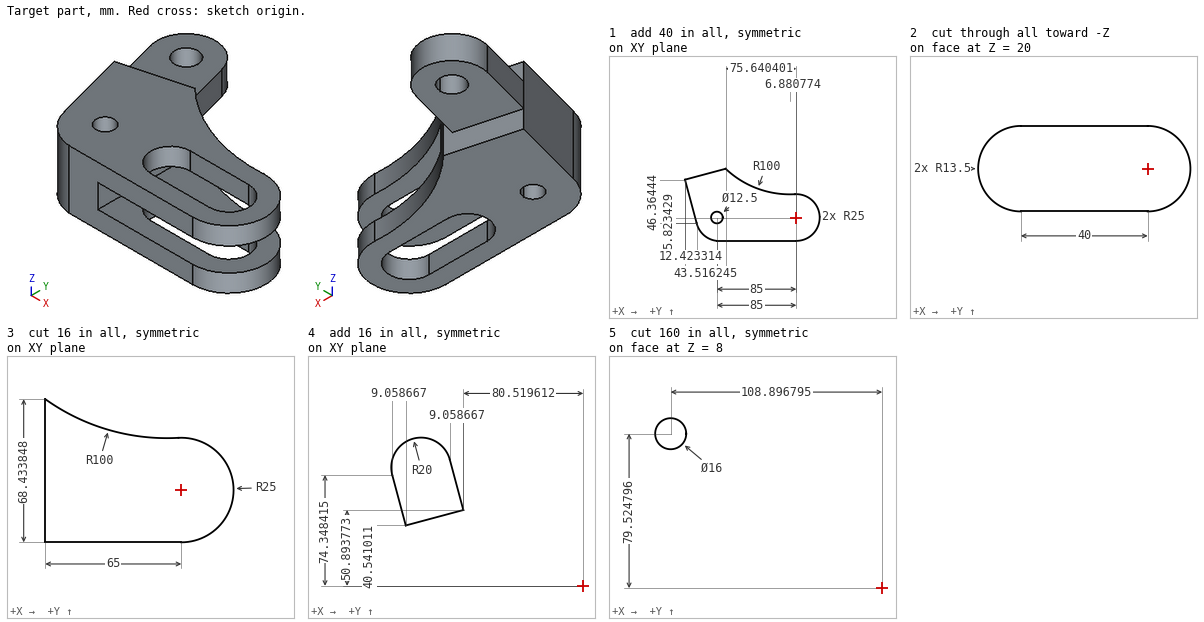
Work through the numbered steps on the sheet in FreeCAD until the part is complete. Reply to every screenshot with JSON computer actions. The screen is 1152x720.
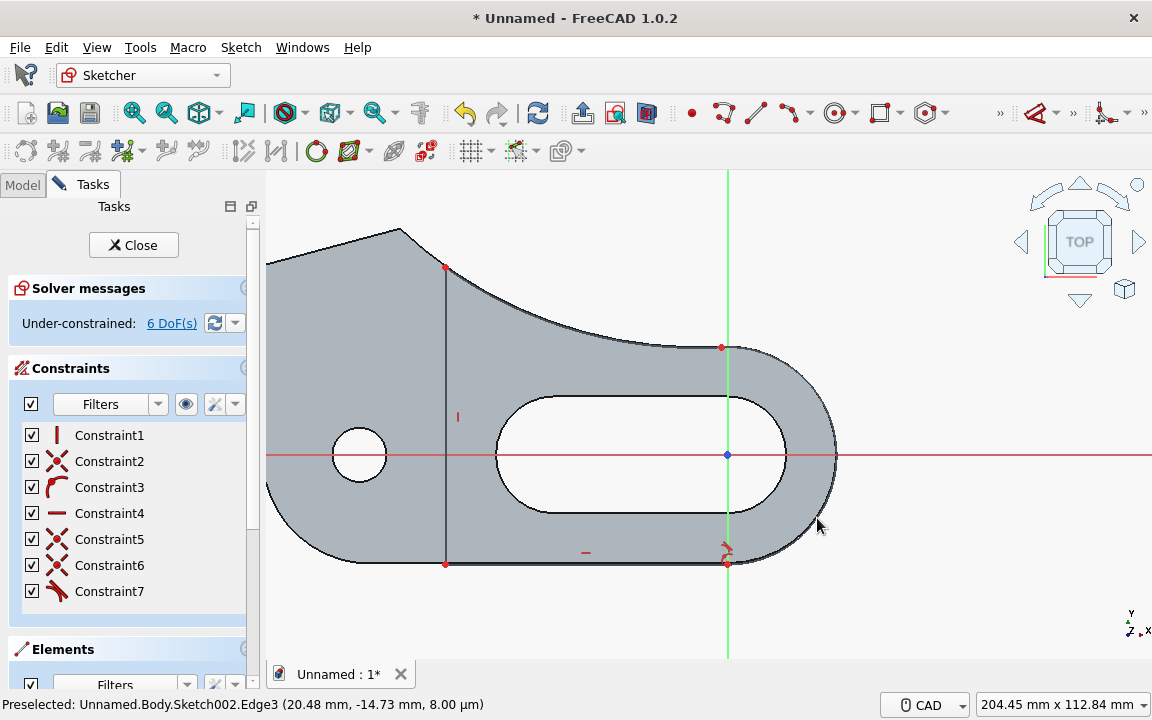
{"action": "left_click", "coordinate": [817, 518]}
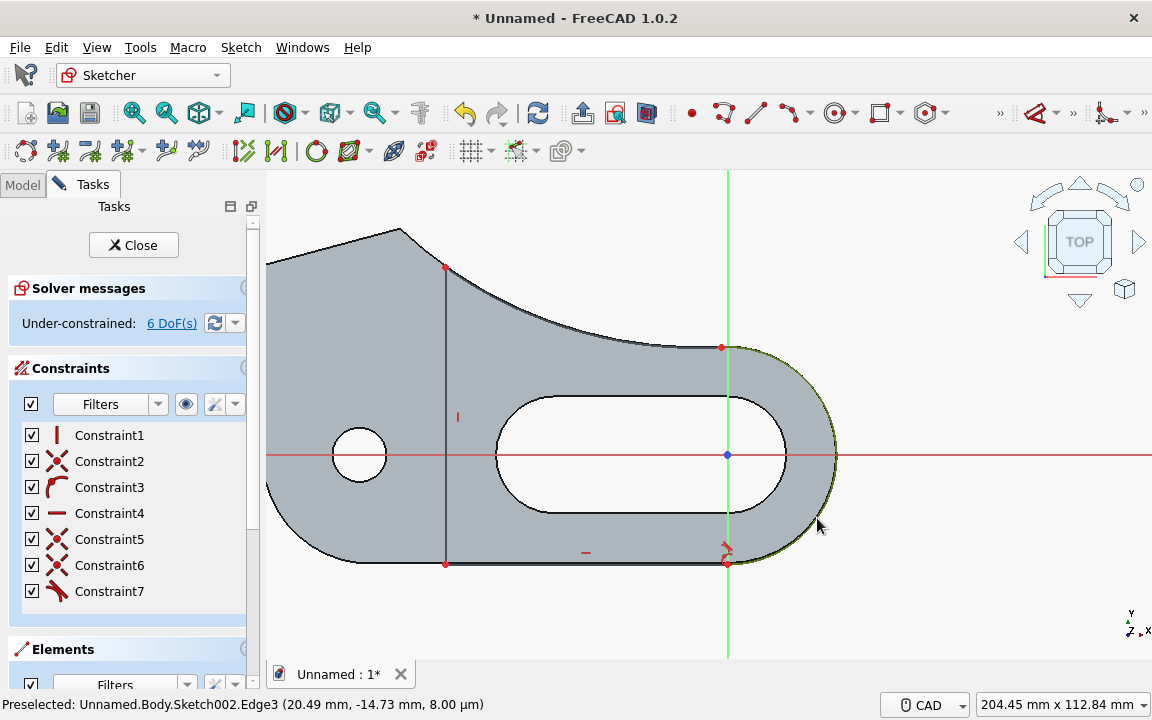
{"action": "left_click", "coordinate": [522, 311]}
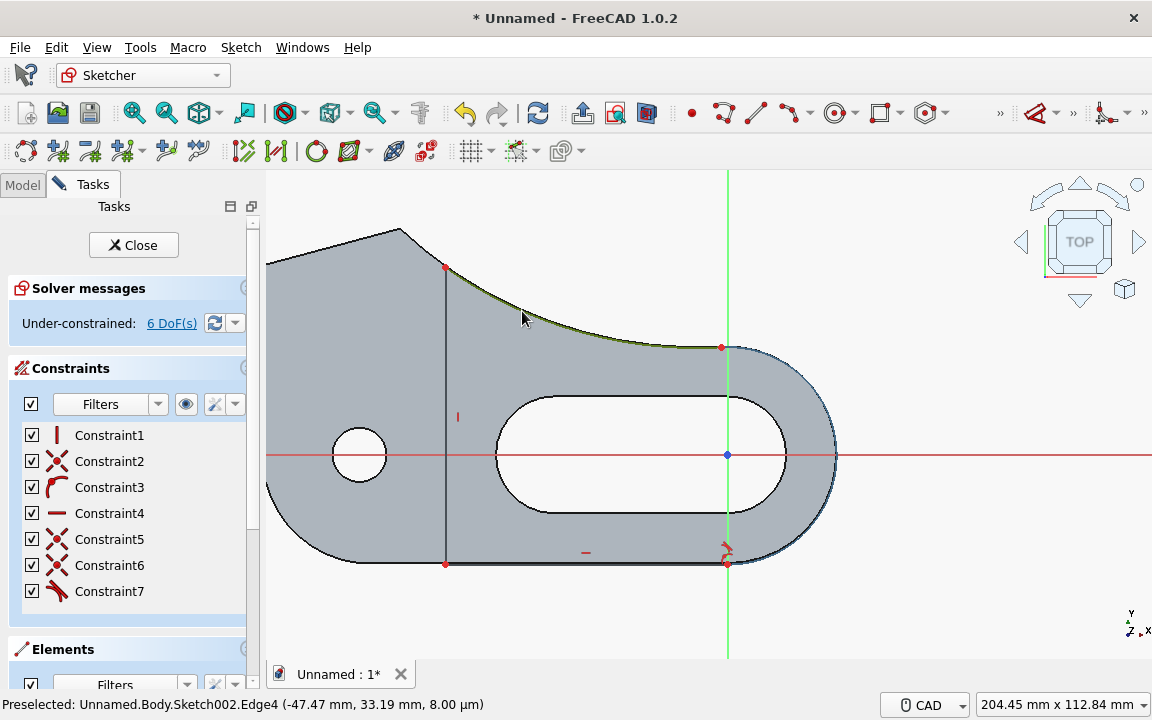
{"action": "key", "text": "t"}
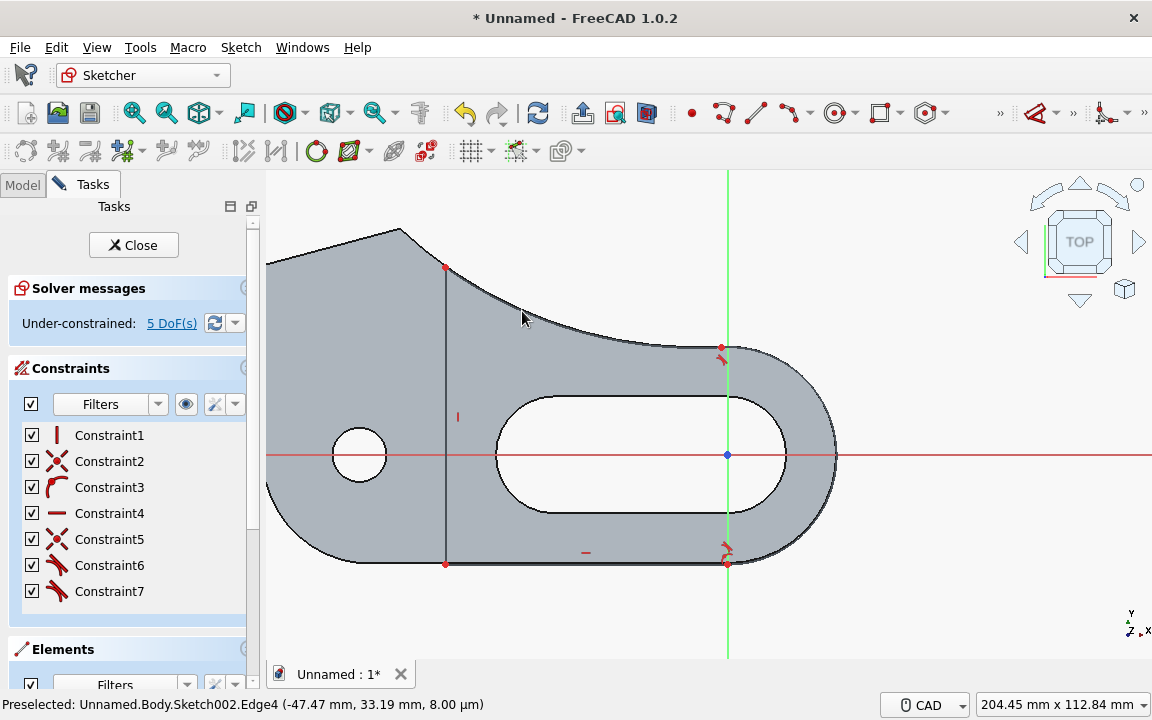
{"action": "left_click", "coordinate": [728, 456]}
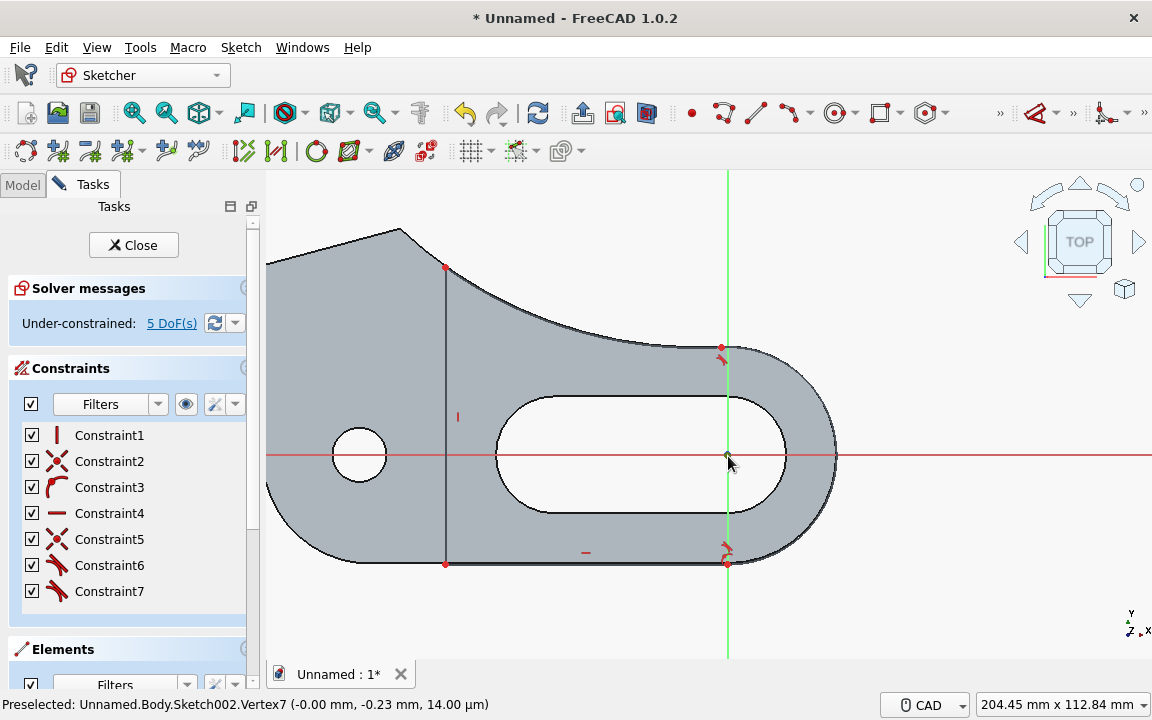
{"action": "left_click", "coordinate": [344, 455]}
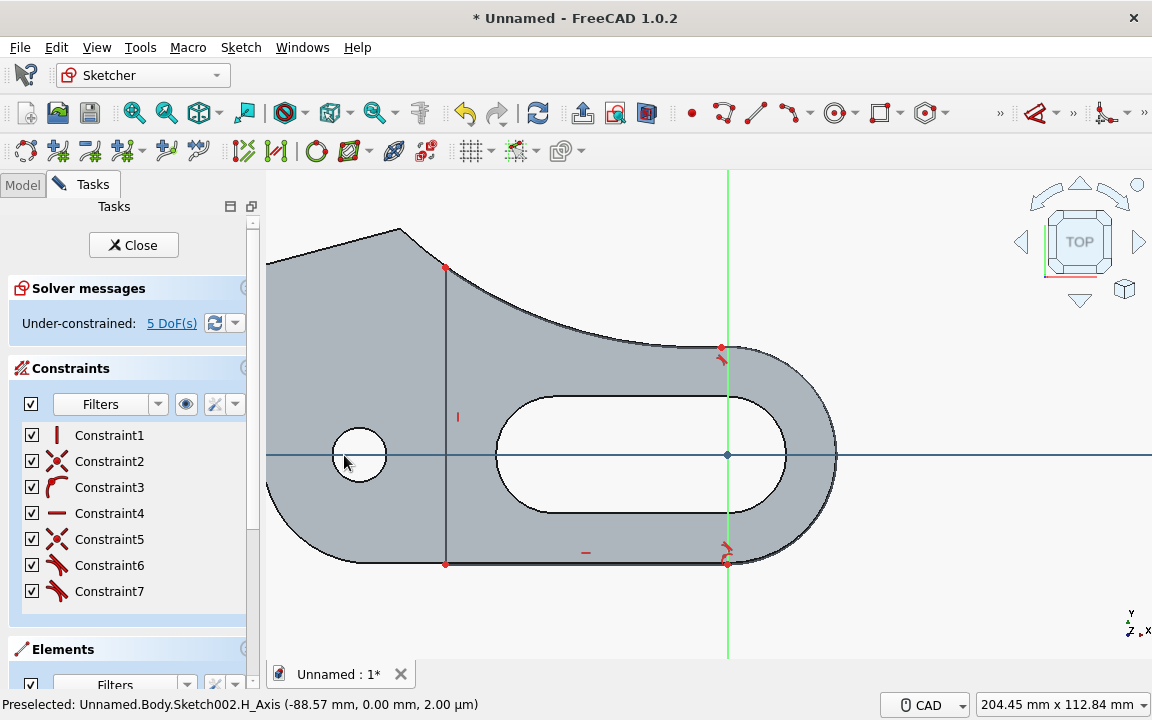
{"action": "key", "text": "c"}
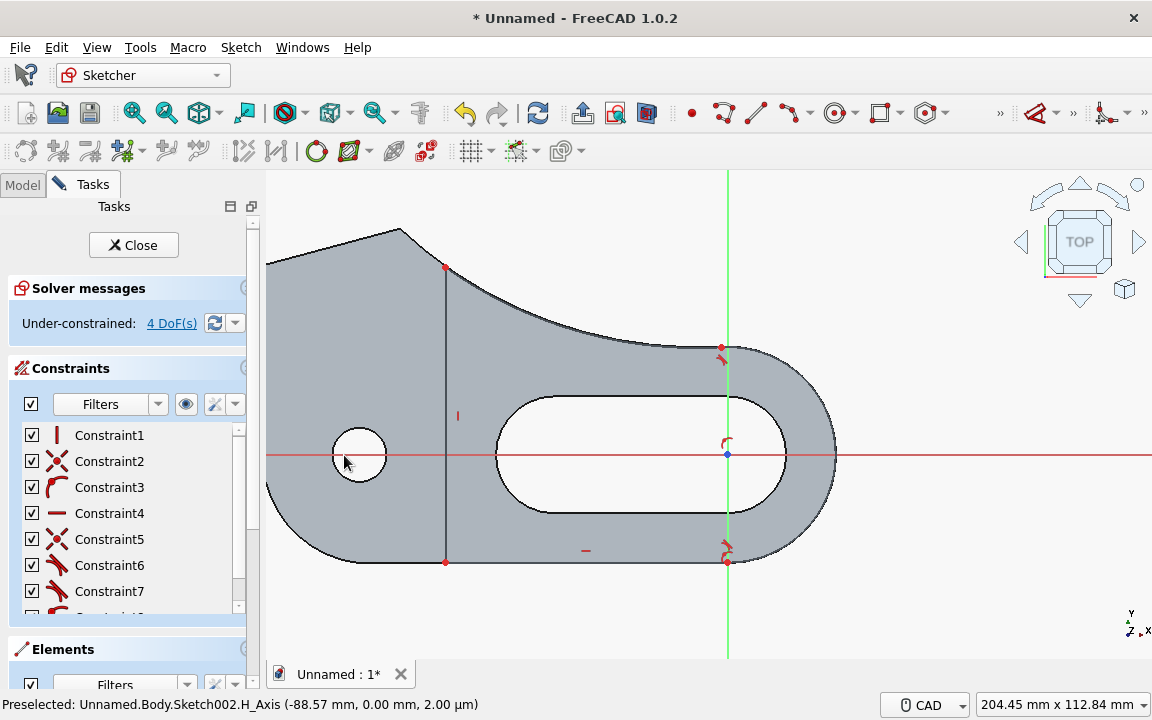
{"action": "left_click", "coordinate": [1036, 114]}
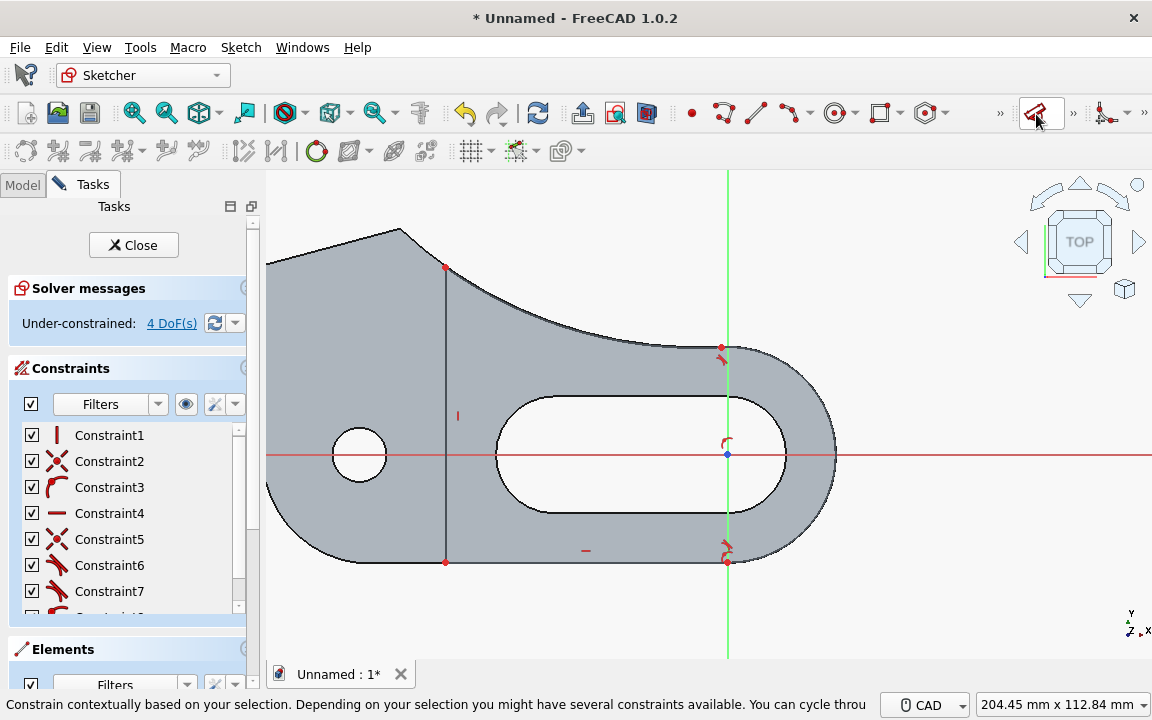
{"action": "left_click", "coordinate": [816, 517]}
{"action": "left_click", "coordinate": [842, 535]}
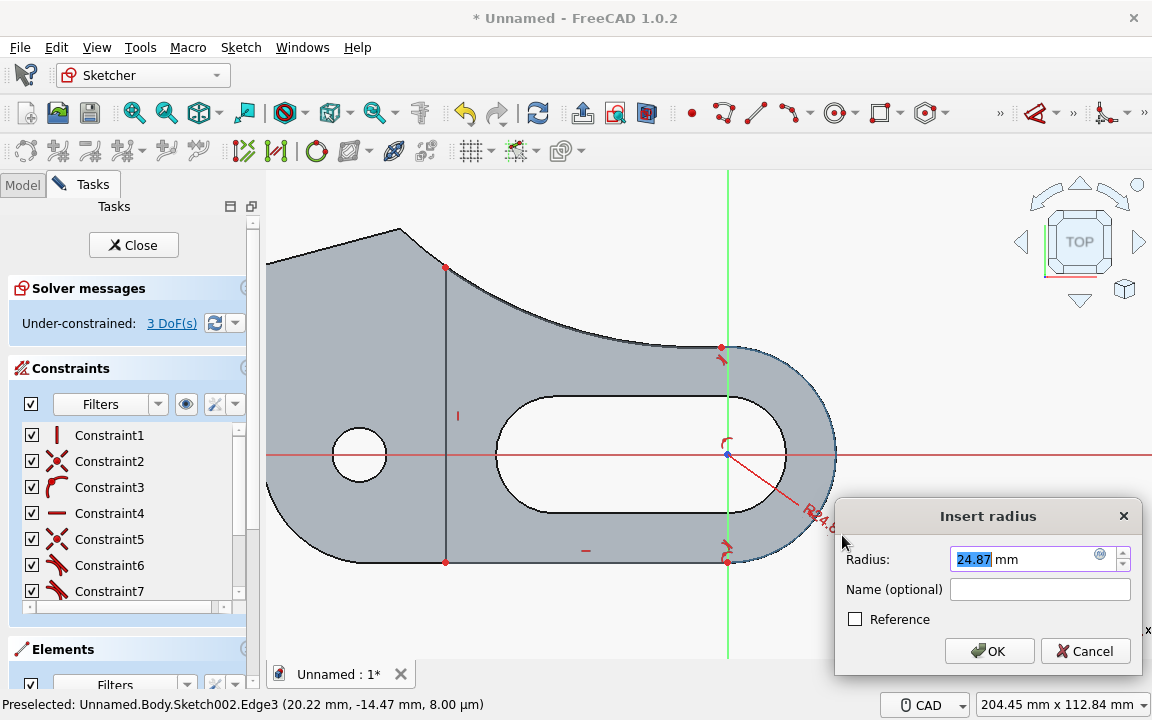
{"action": "type", "text": "25"}
{"action": "key", "text": "Return"}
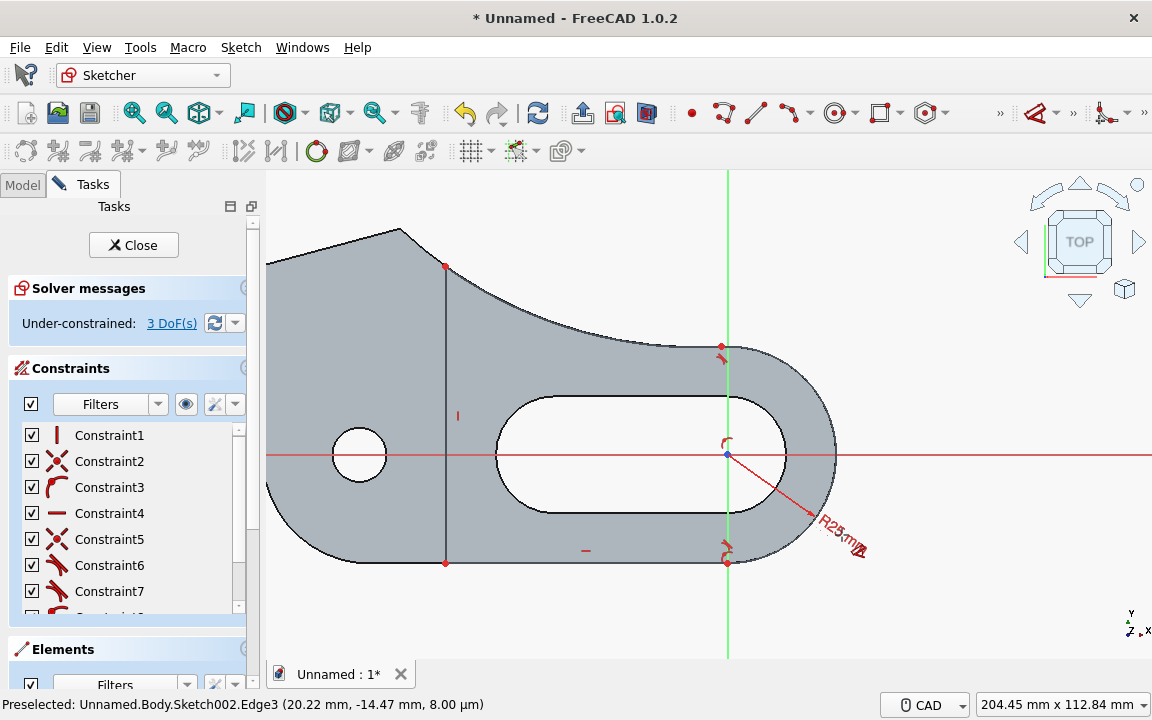
{"action": "left_click", "coordinate": [522, 310]}
{"action": "left_click", "coordinate": [509, 339]}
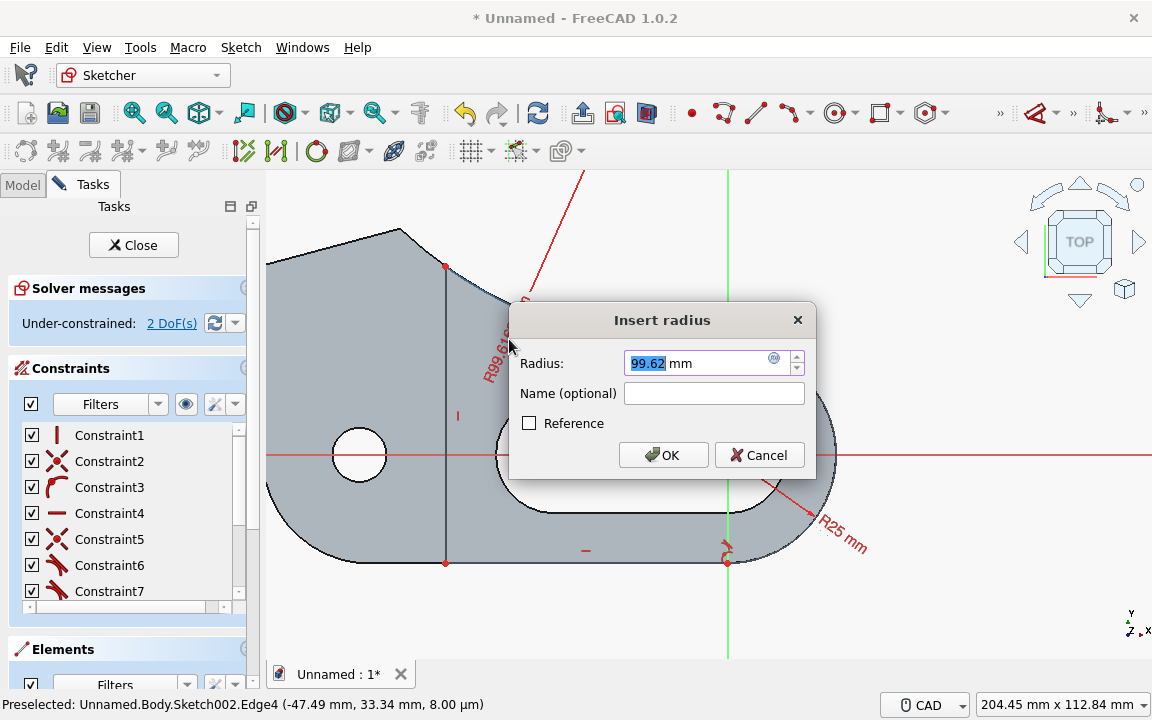
{"action": "type", "text": "100"}
{"action": "key", "text": "Return"}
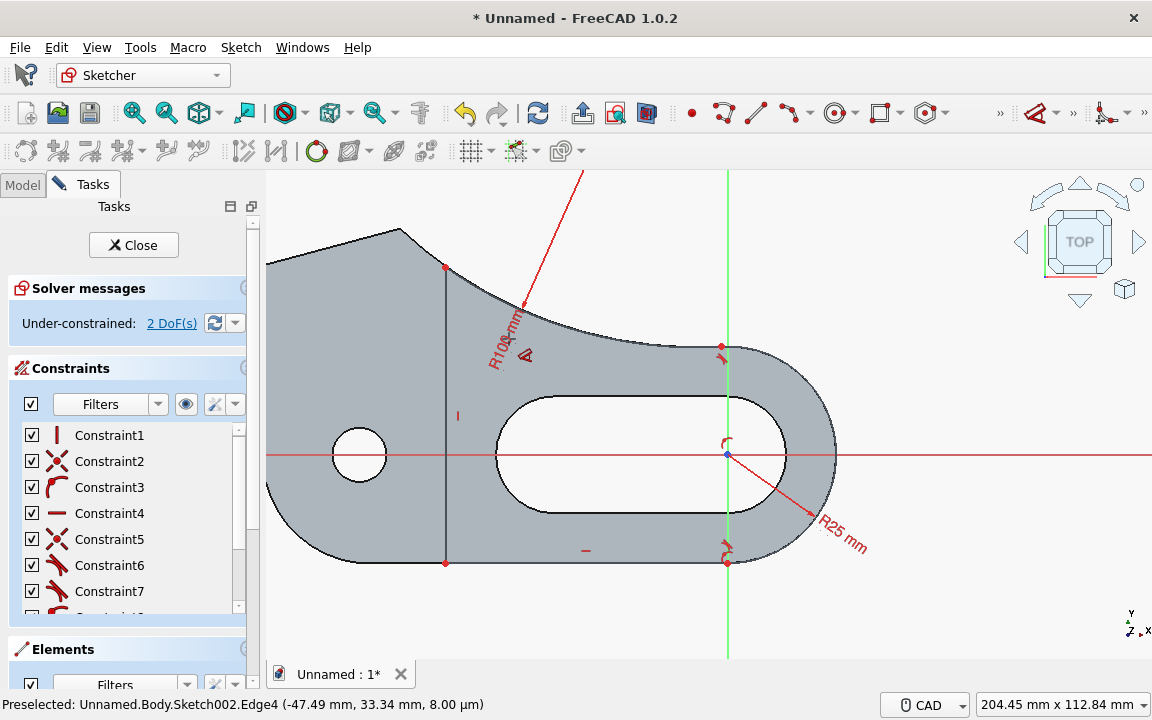
{"action": "left_click", "coordinate": [530, 563]}
{"action": "left_click", "coordinate": [587, 597]}